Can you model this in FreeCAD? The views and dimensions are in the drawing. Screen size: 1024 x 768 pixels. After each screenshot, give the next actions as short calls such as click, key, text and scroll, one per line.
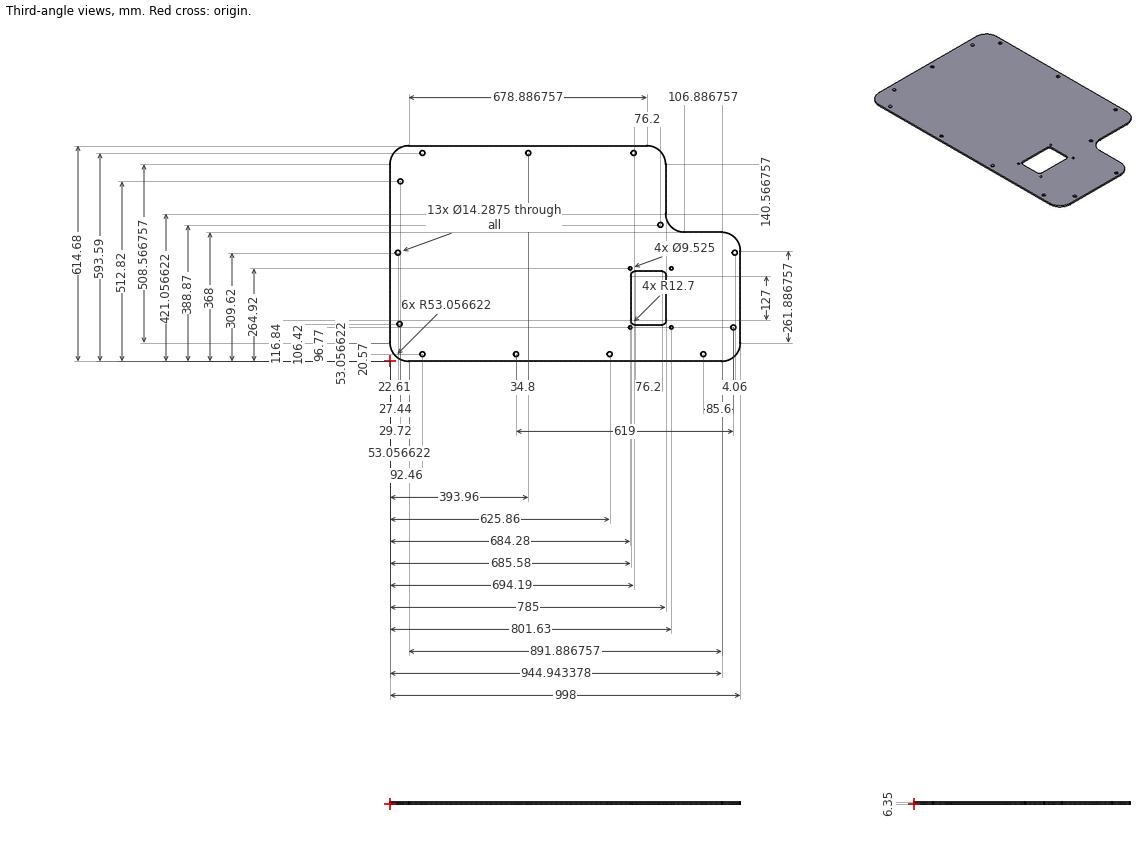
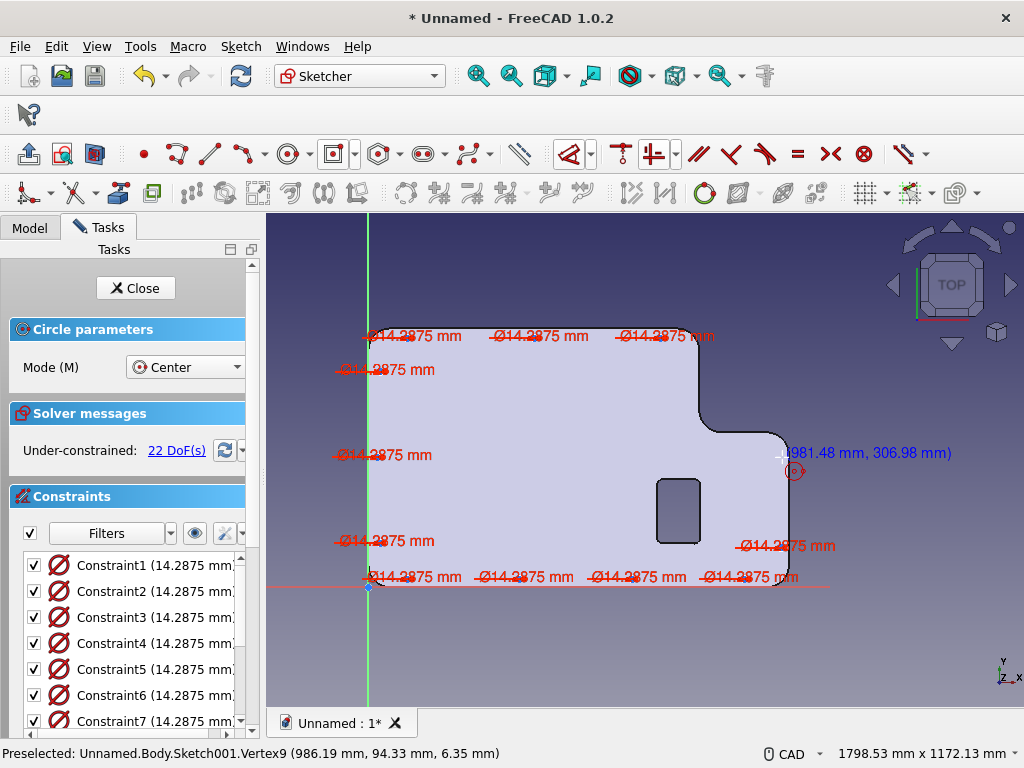
click(782, 457)
move(784, 455)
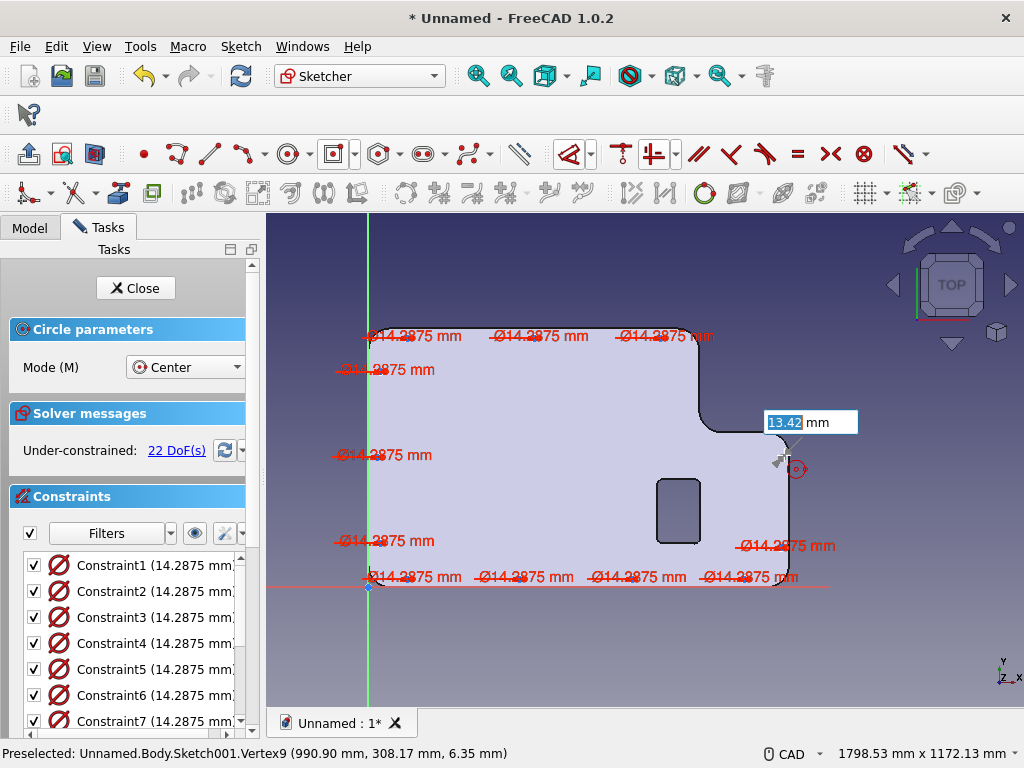
text(14.2875)
key(Return)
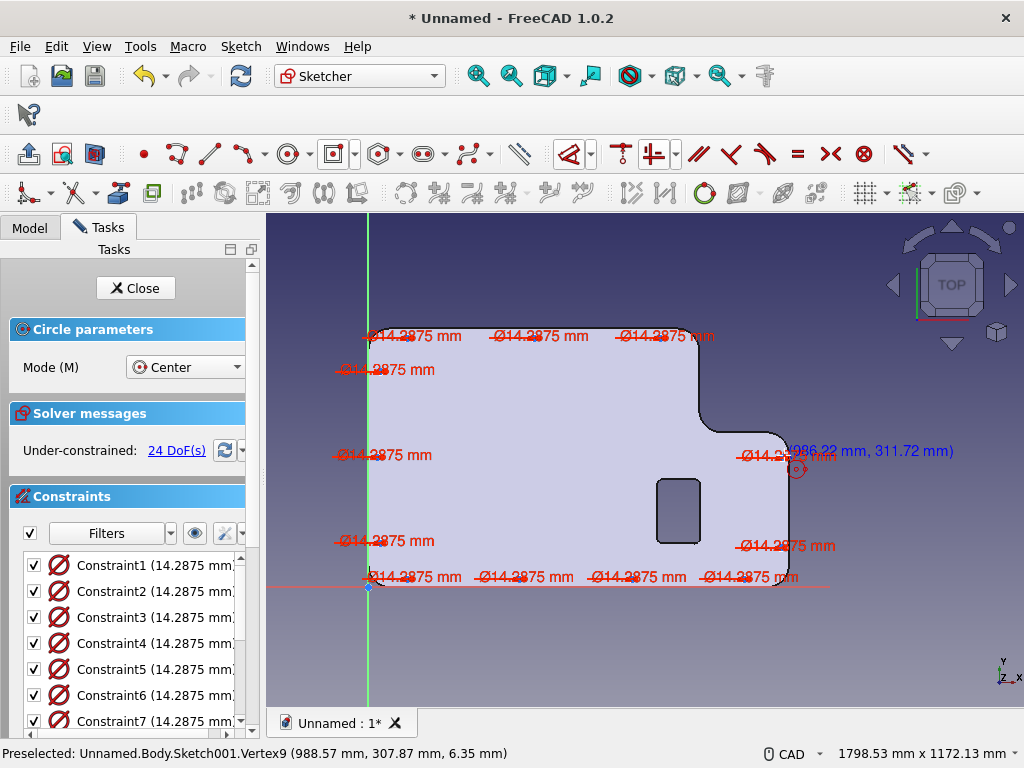
scroll(693, 423, up, 11)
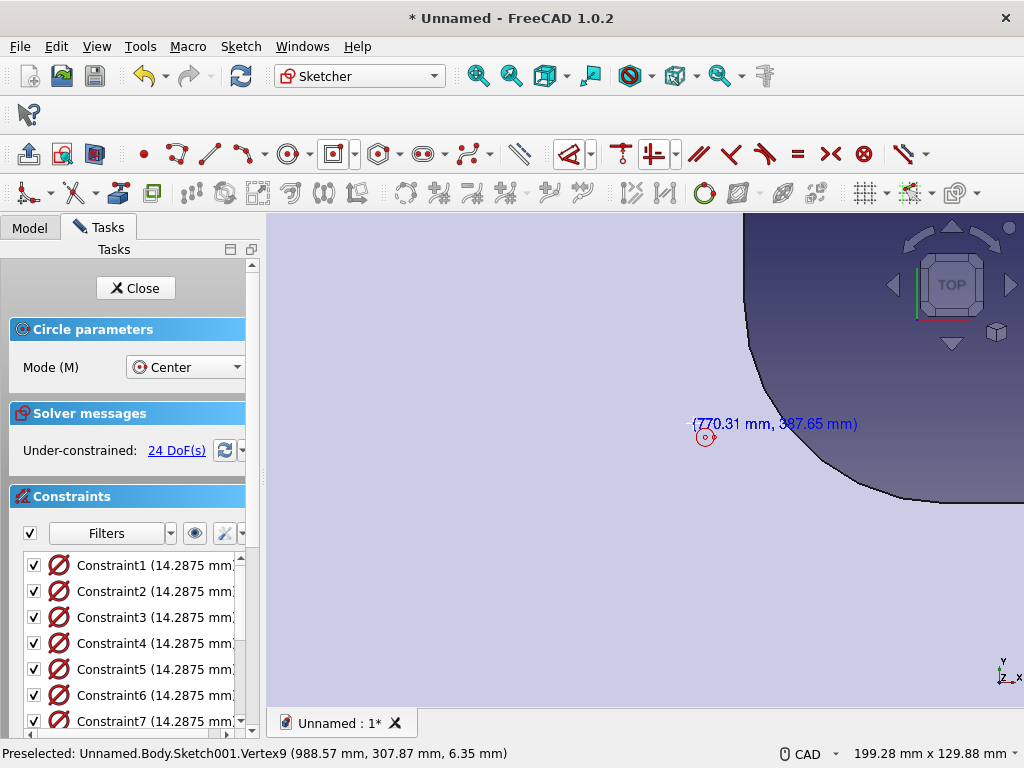
scroll(693, 423, down, 11)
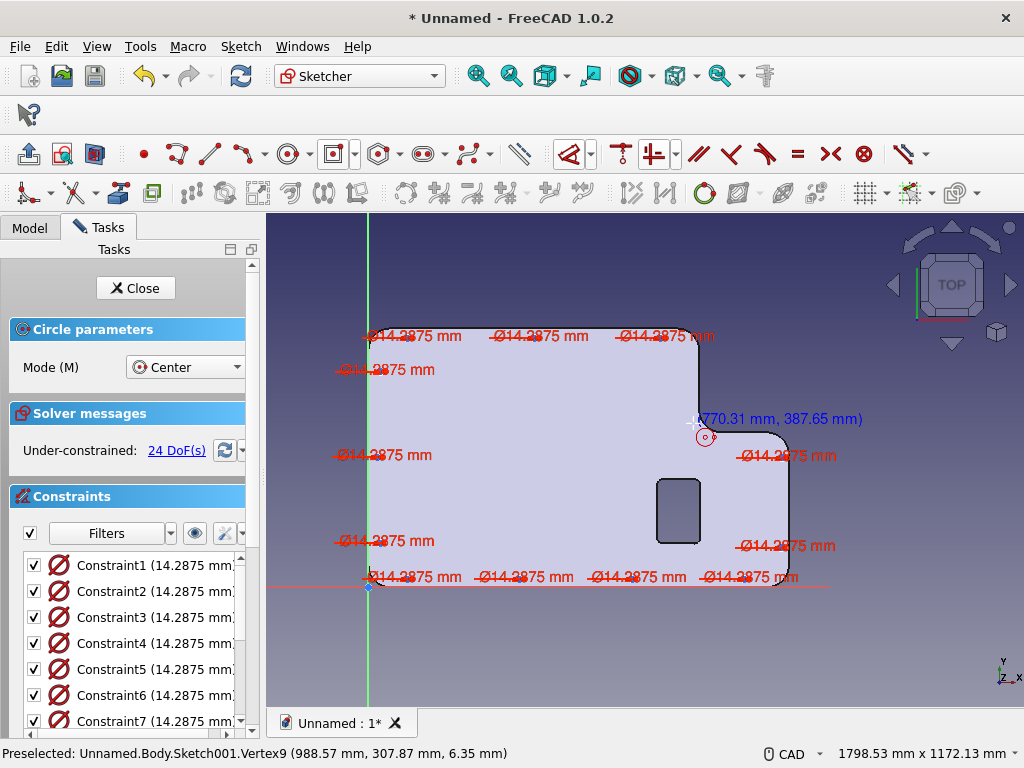
click(693, 423)
move(695, 421)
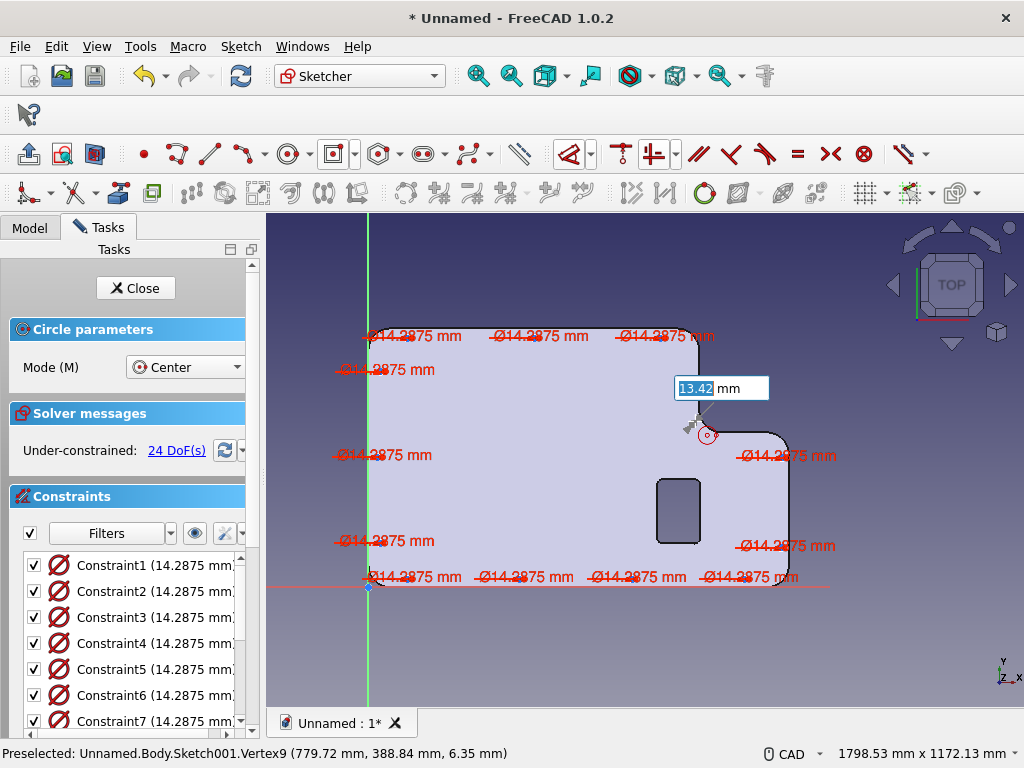
text(14.2875)
key(Return)
key(Escape)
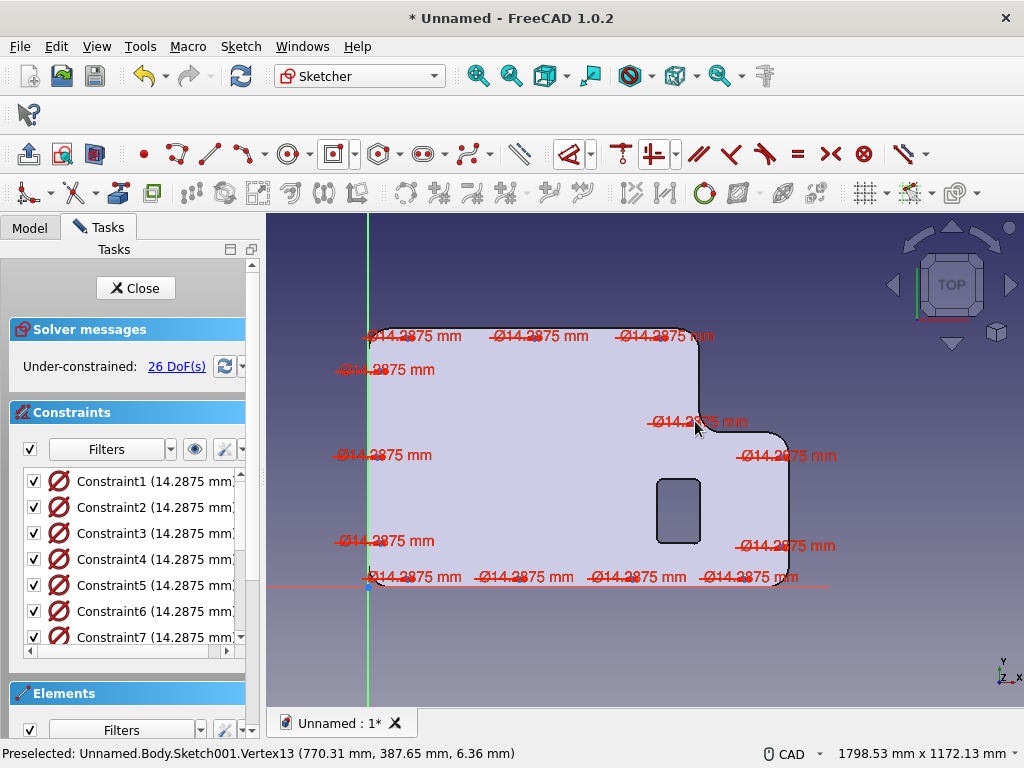
click(520, 579)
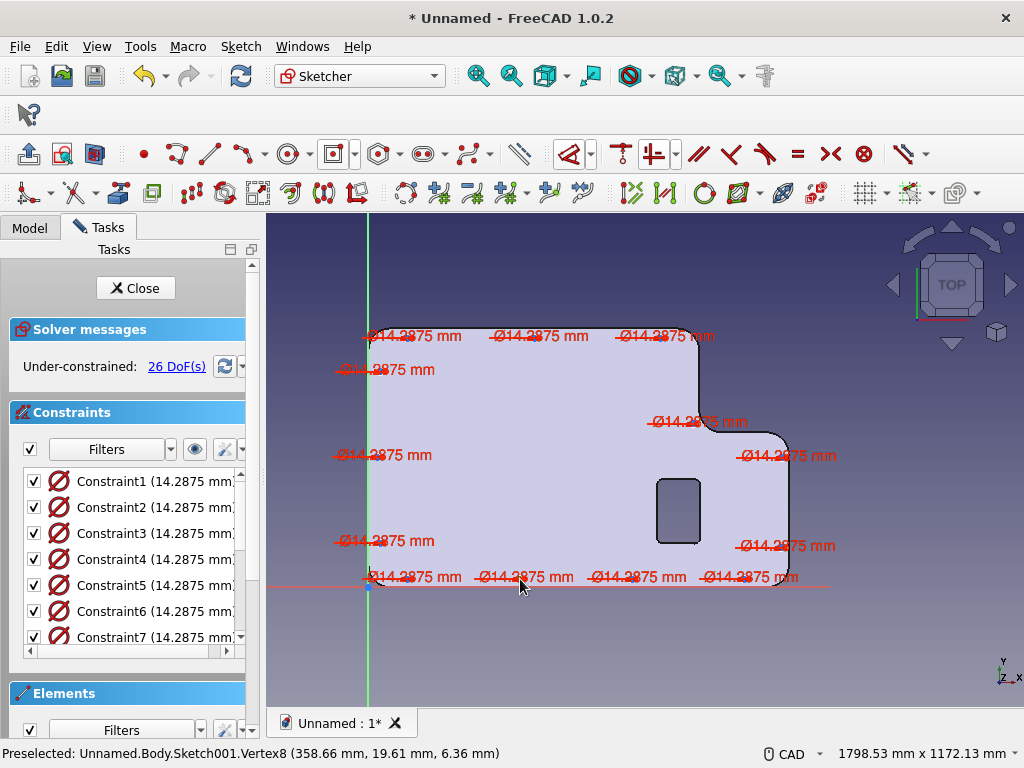
click(781, 548)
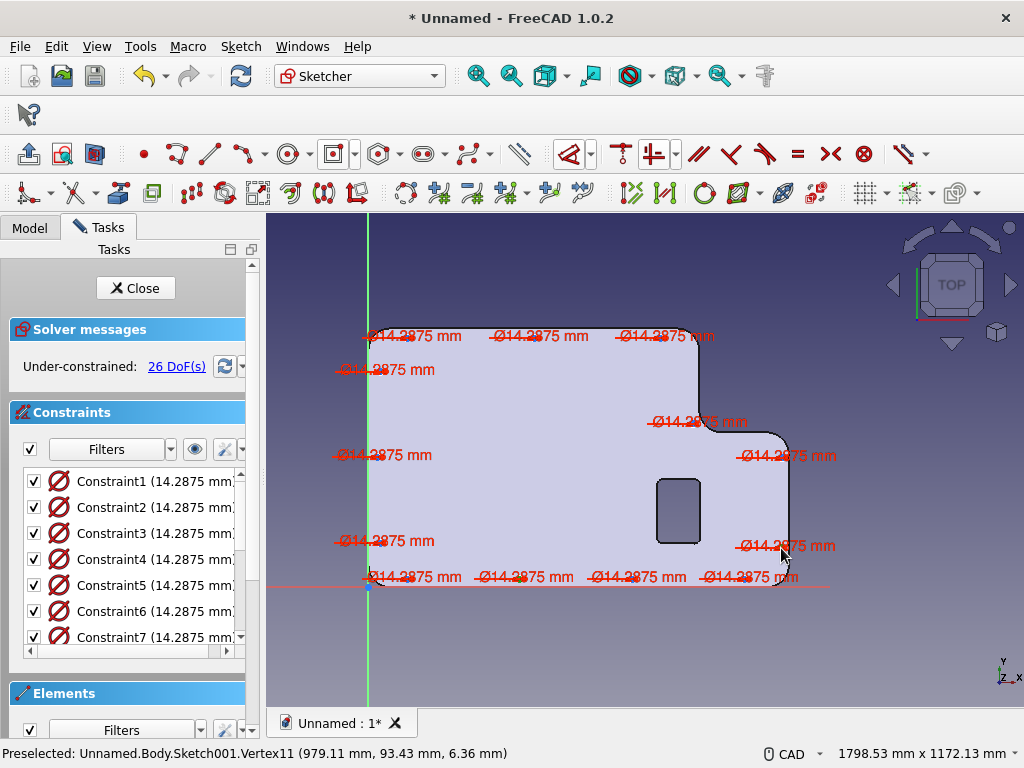
click(590, 154)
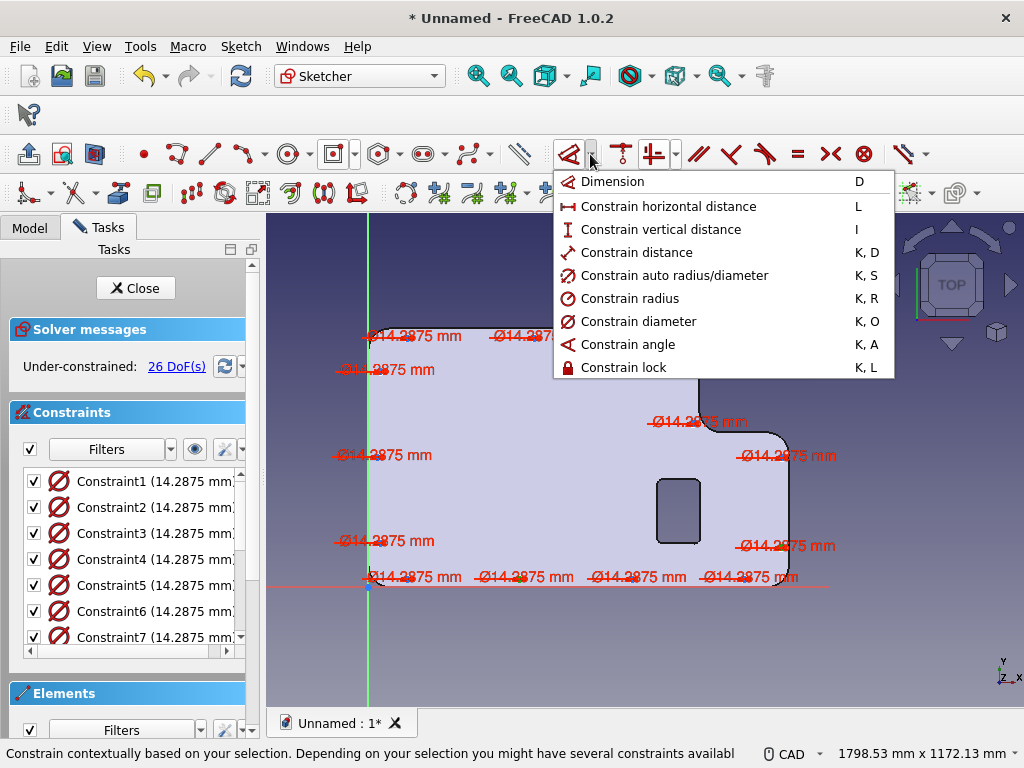
click(724, 206)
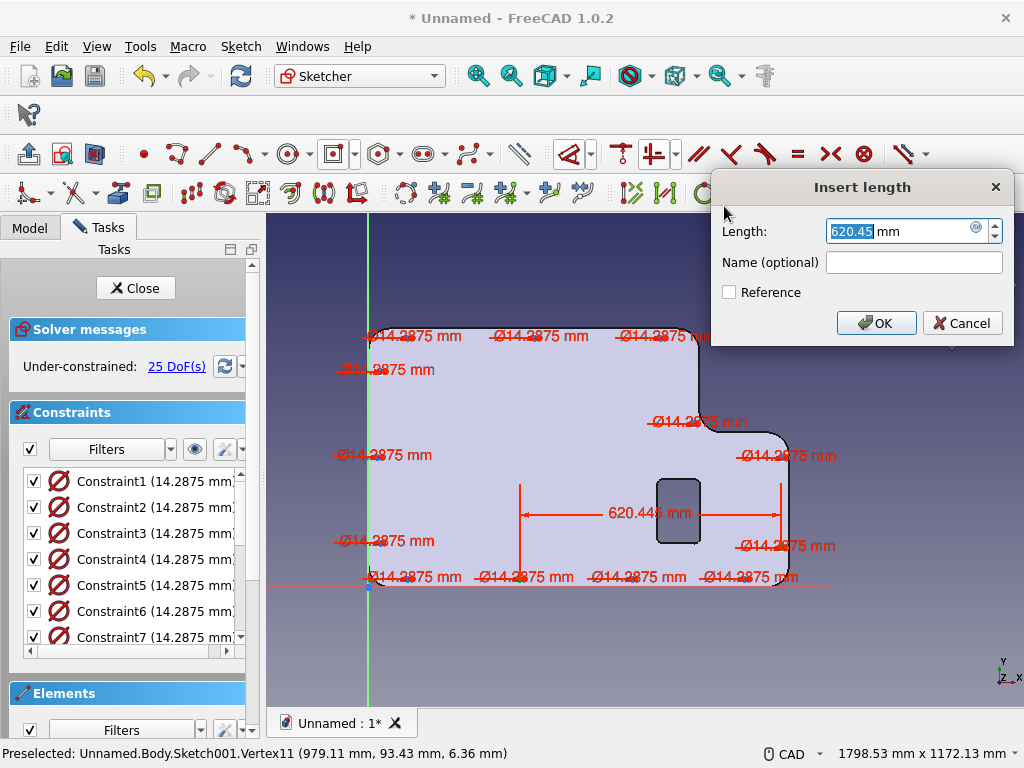
text(619)
key(Return)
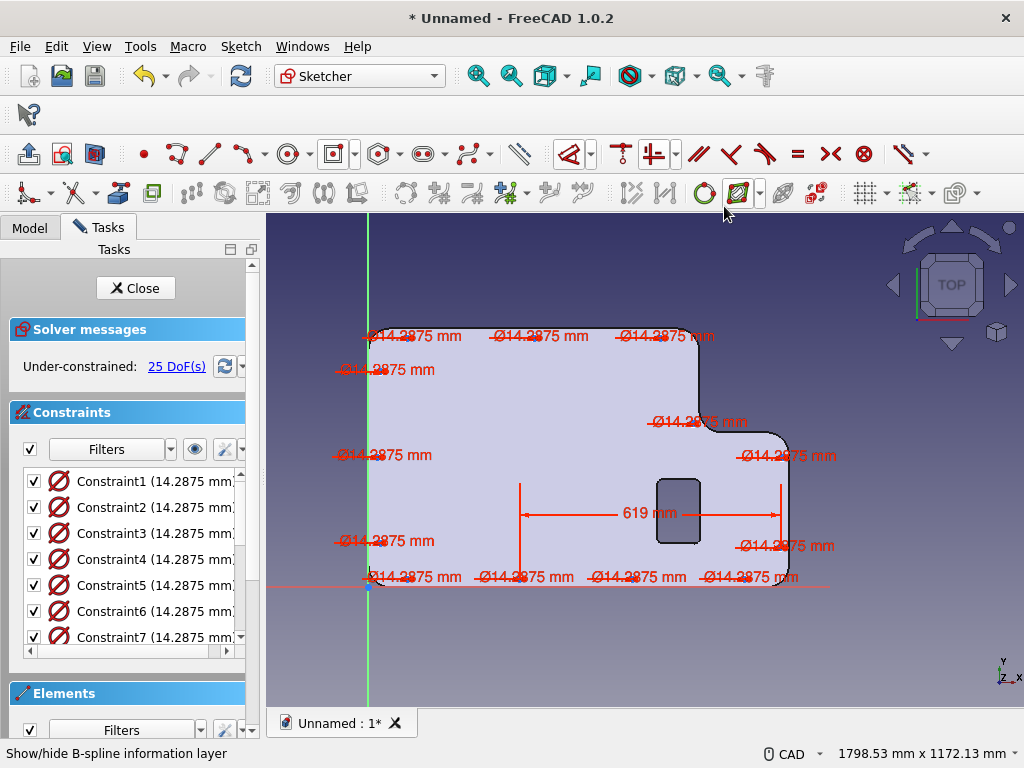
scroll(378, 457, up, 8)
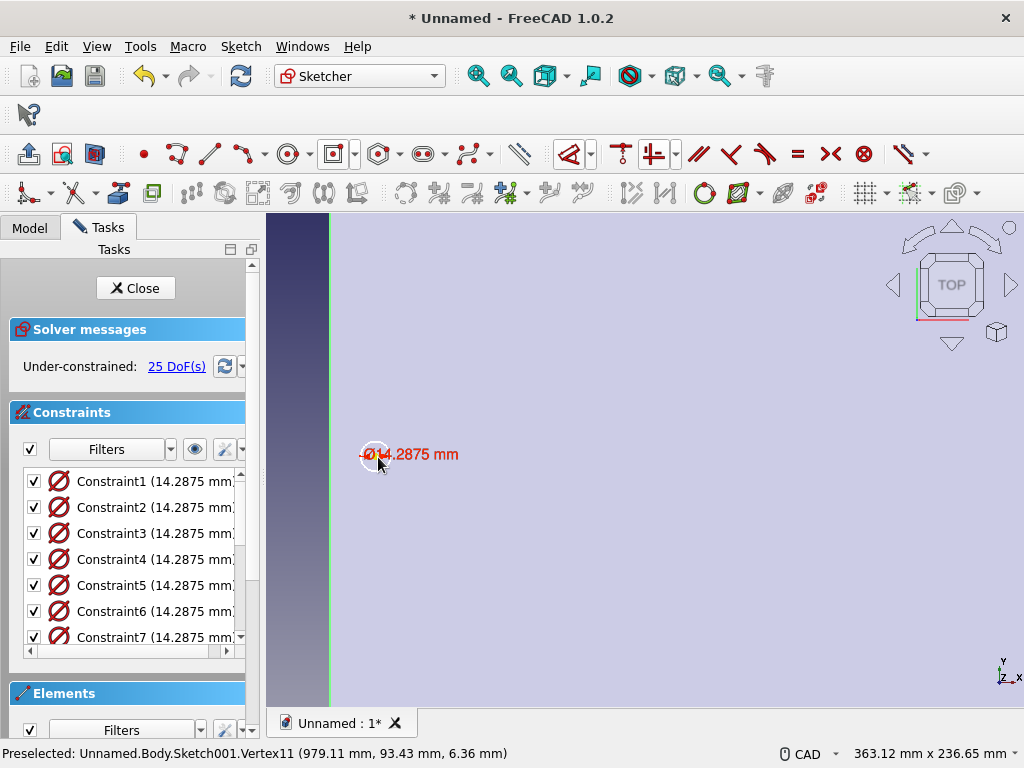
click(376, 456)